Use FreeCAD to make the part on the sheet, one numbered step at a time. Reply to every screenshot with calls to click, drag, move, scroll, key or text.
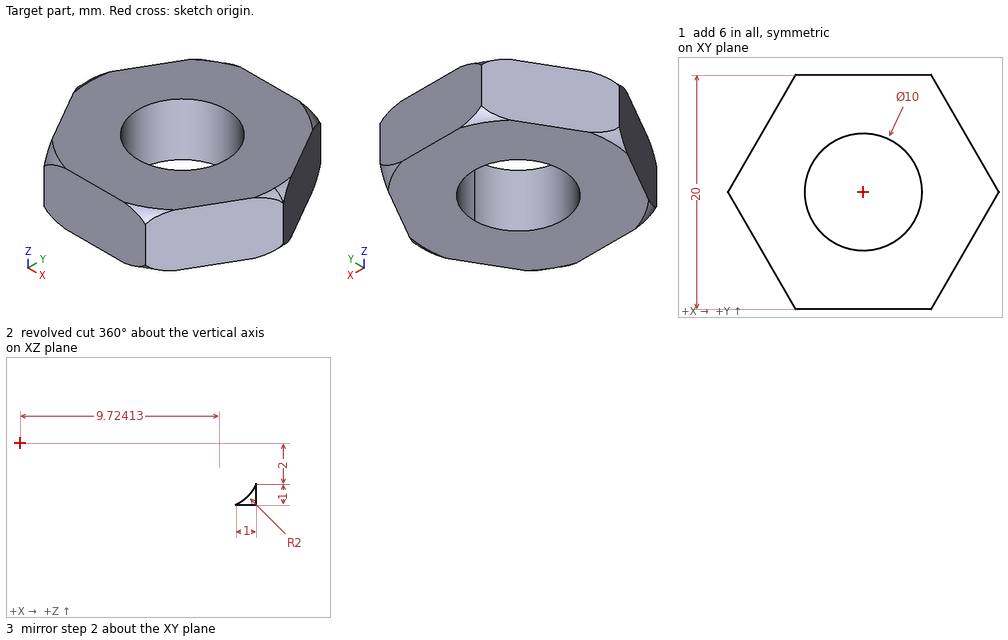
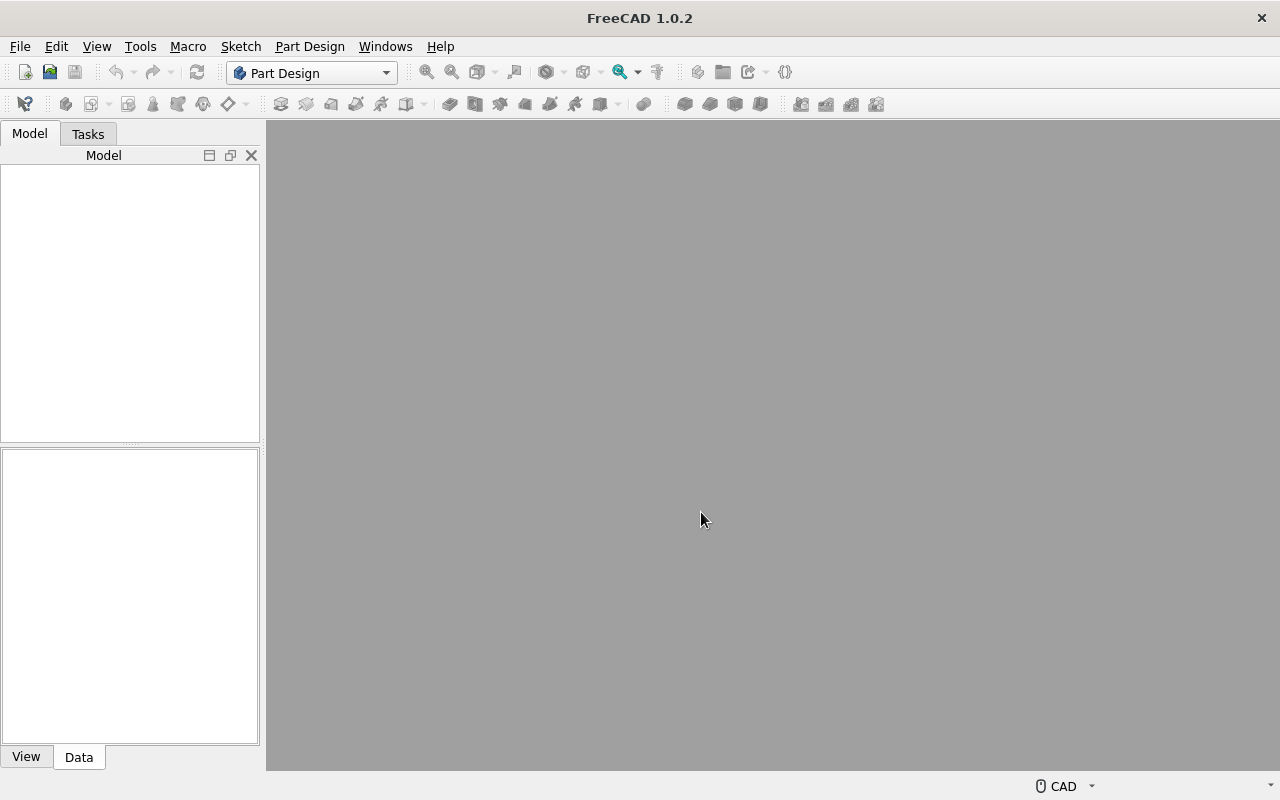
click(25, 72)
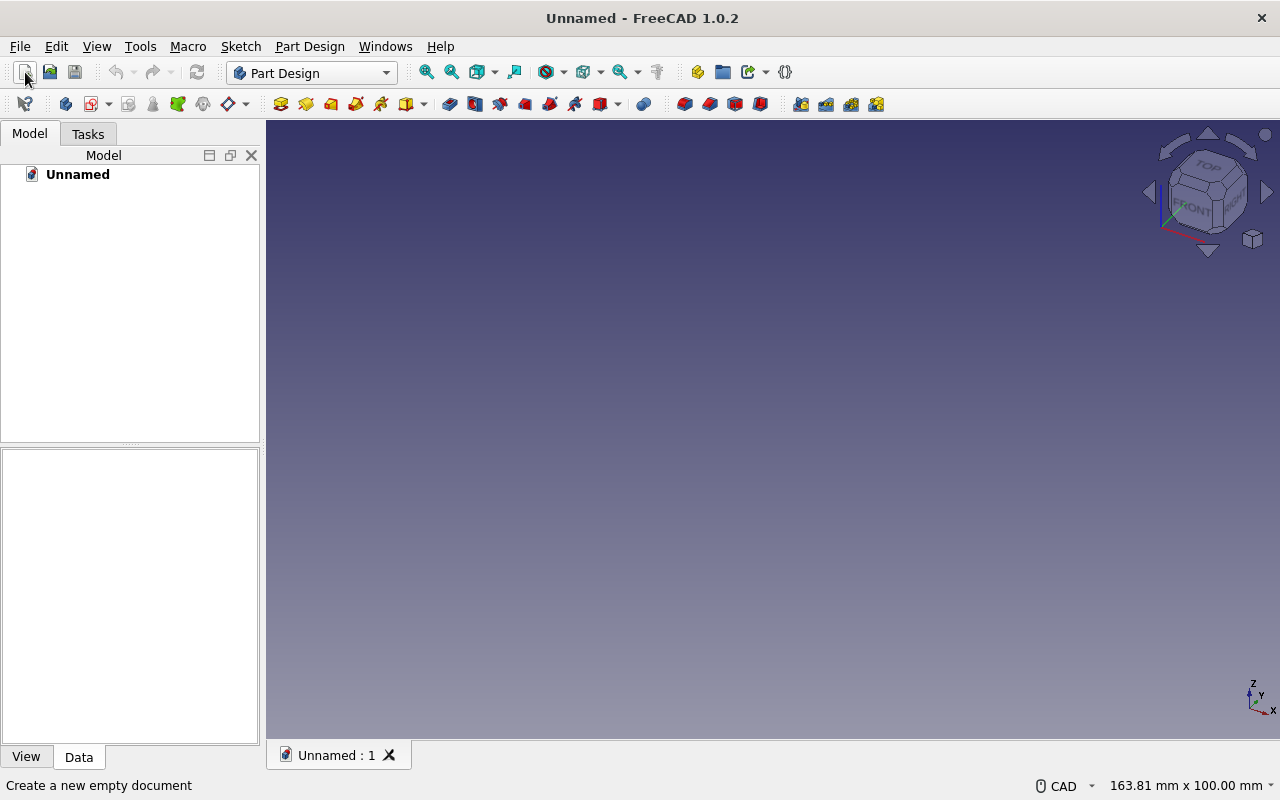
click(90, 104)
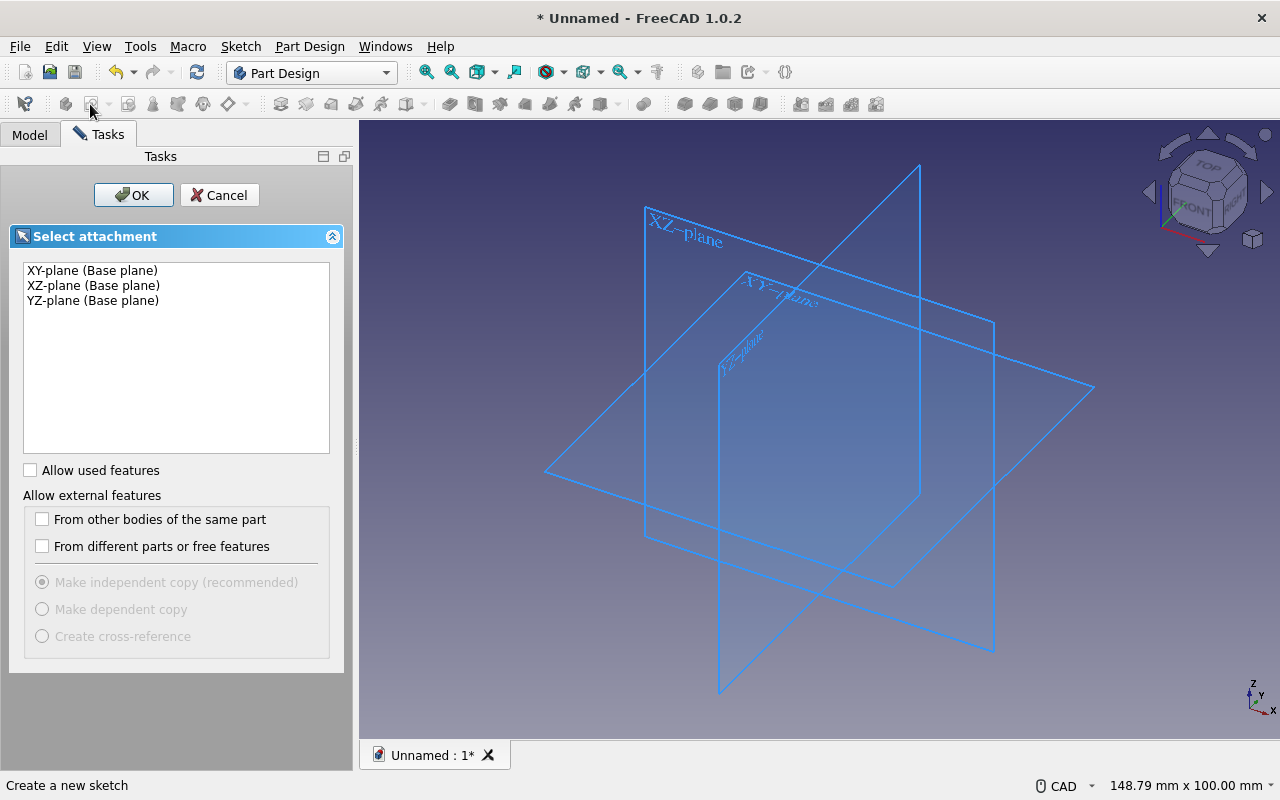
click(84, 270)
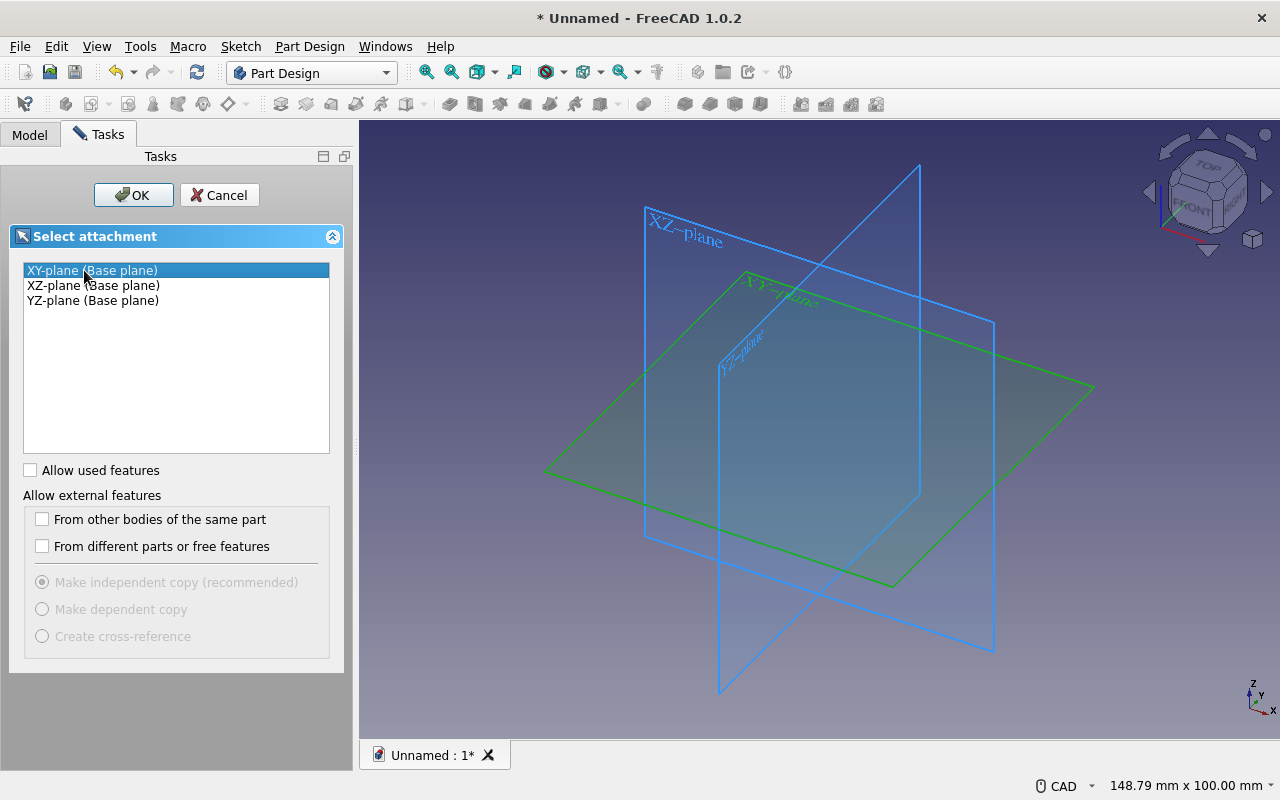
click(134, 195)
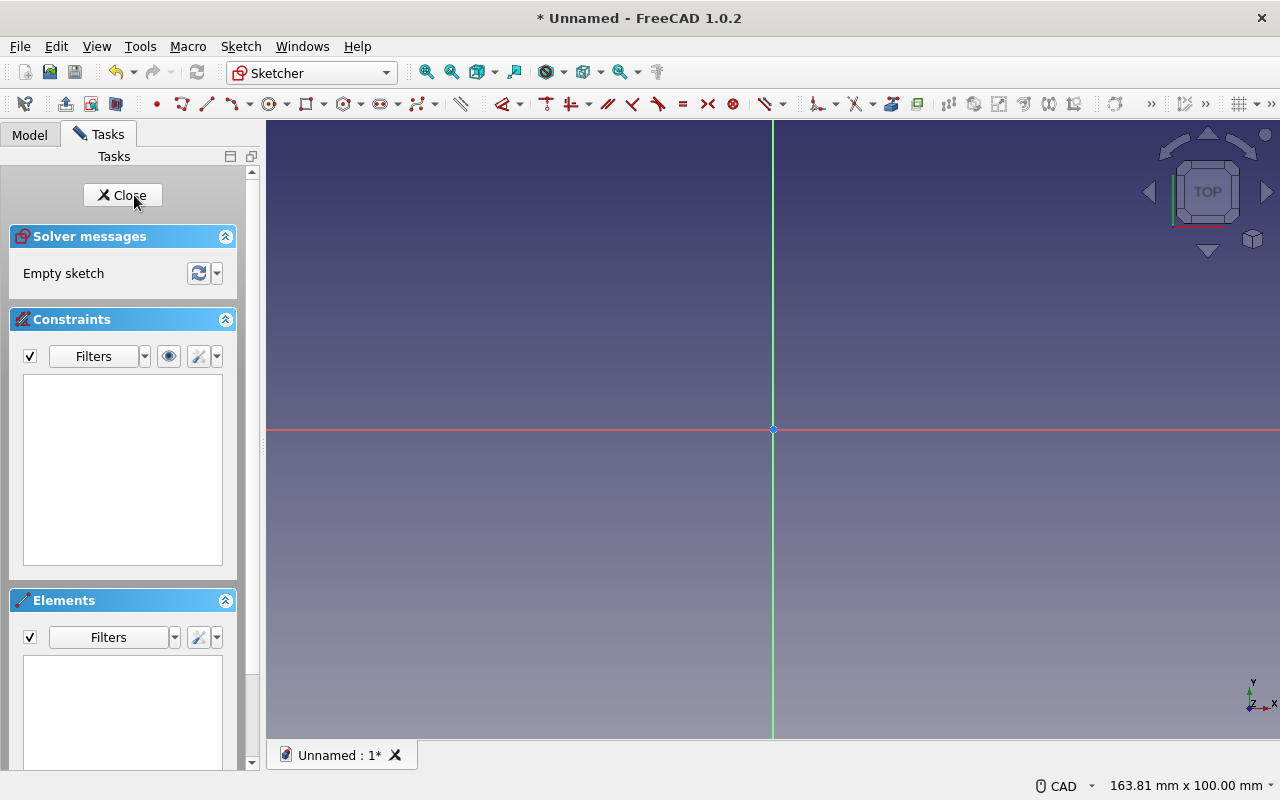
scroll(803, 430, up, 6)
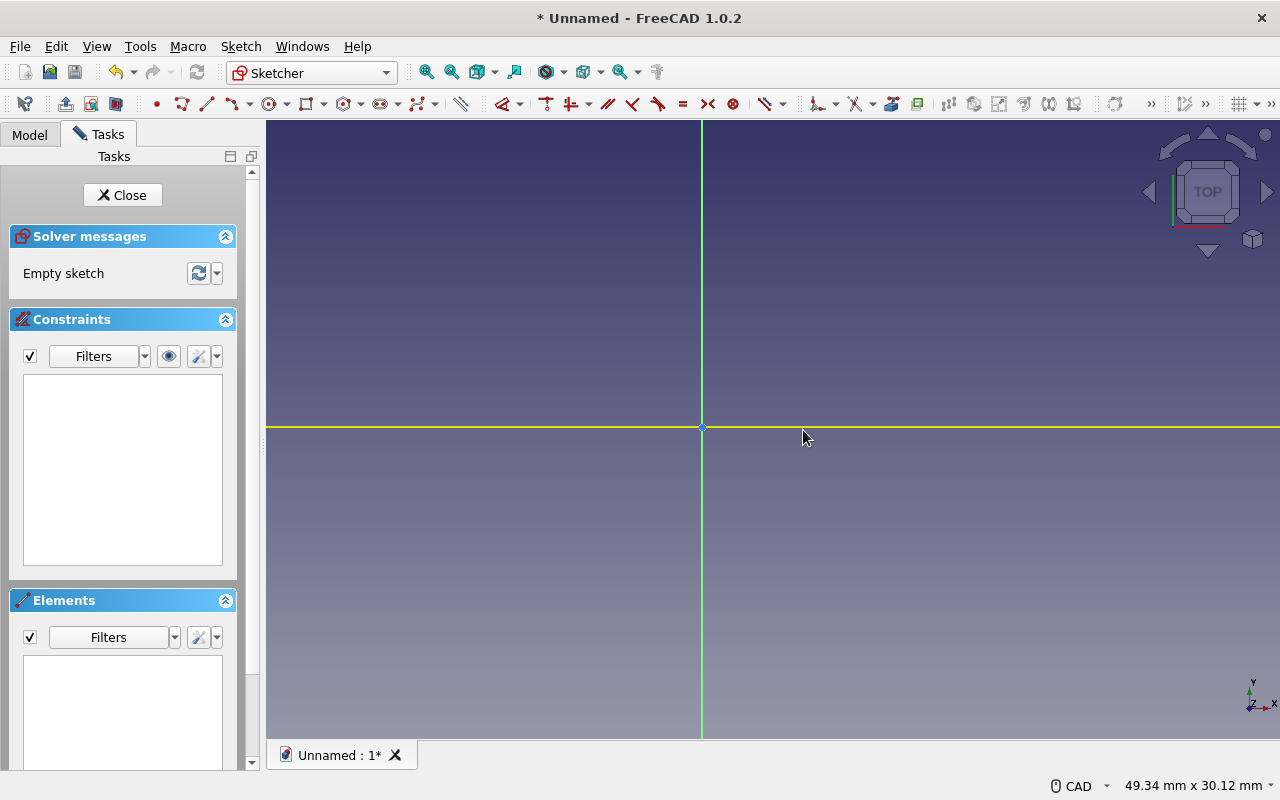
key(g)
key(p)
key(6)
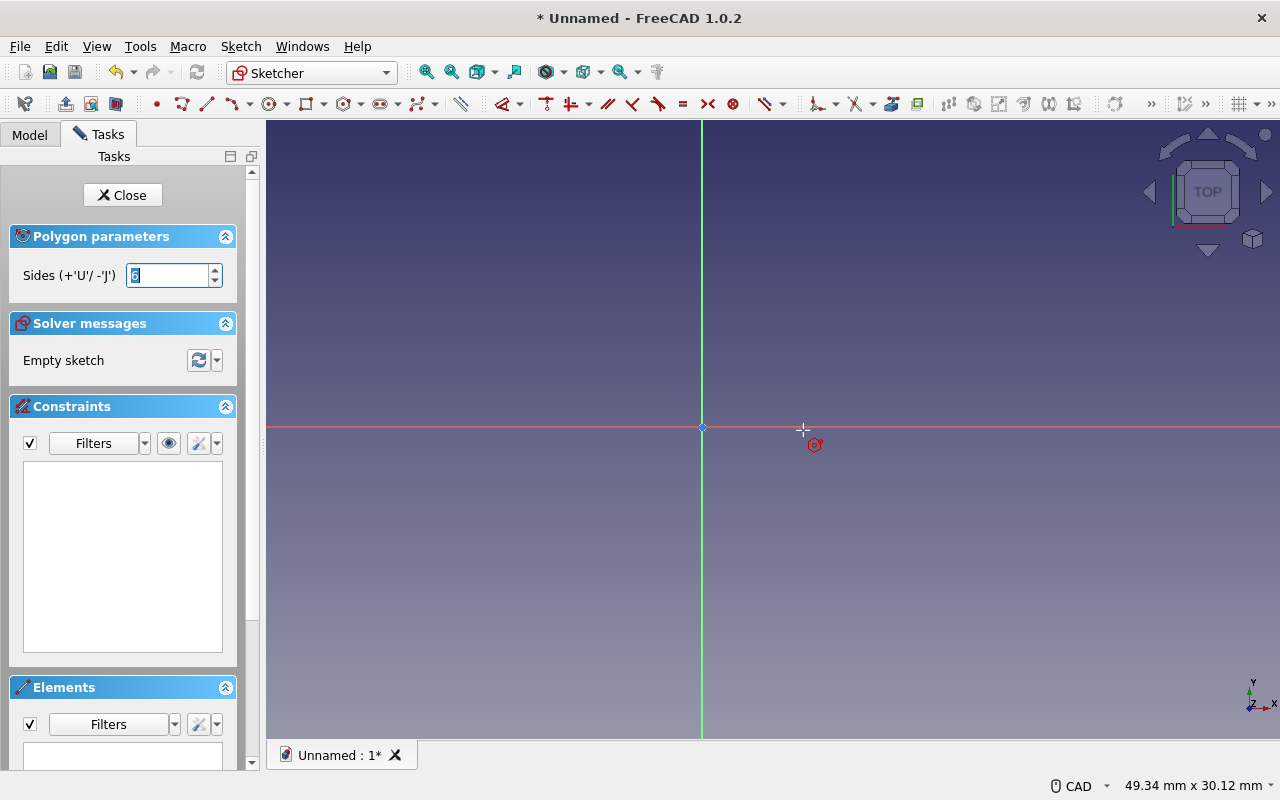
click(702, 427)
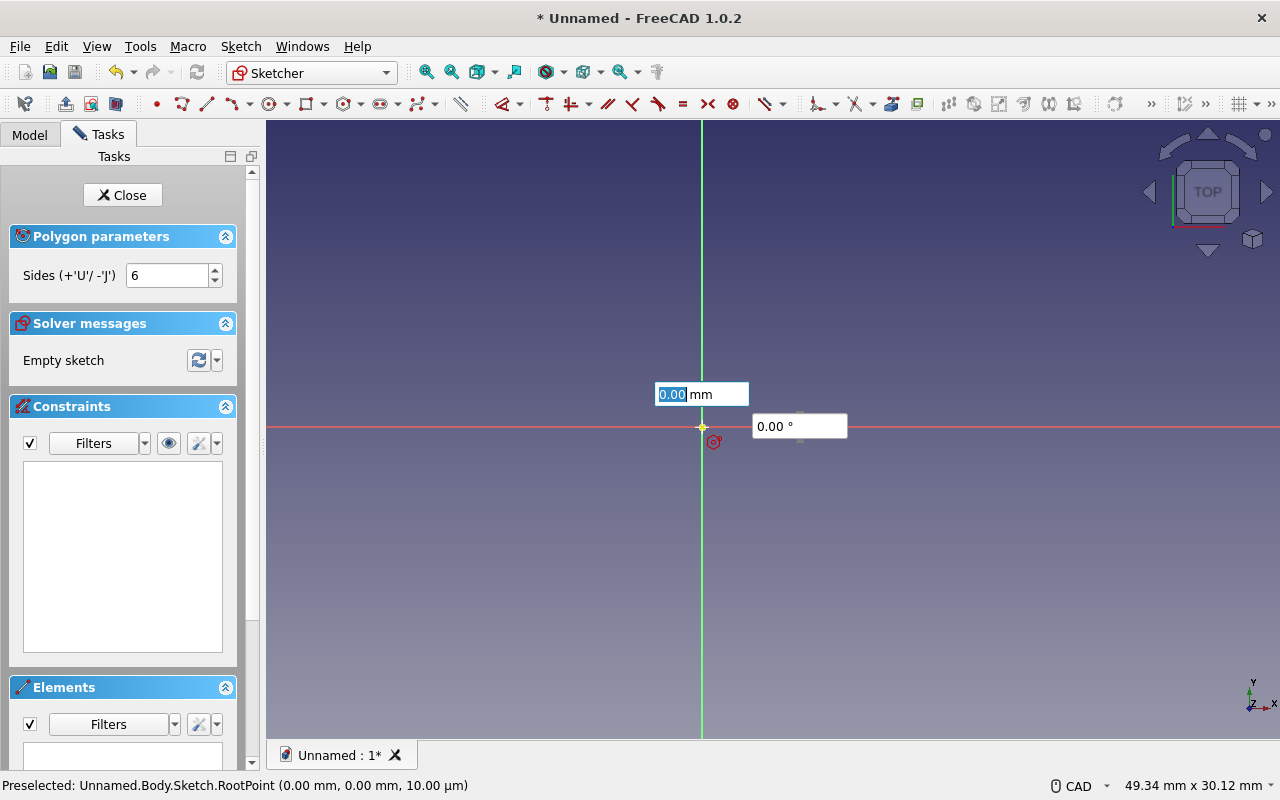
click(939, 427)
right_click(939, 427)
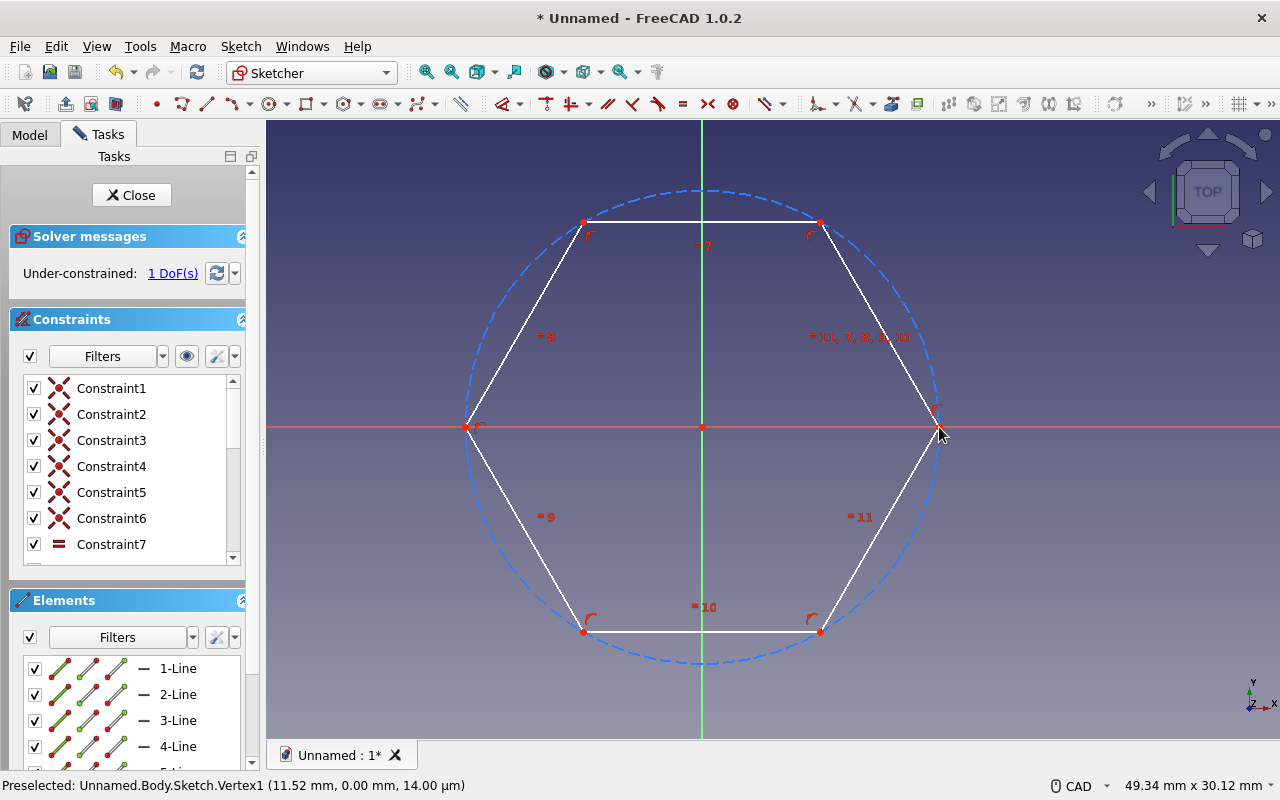
key(g)
key(c)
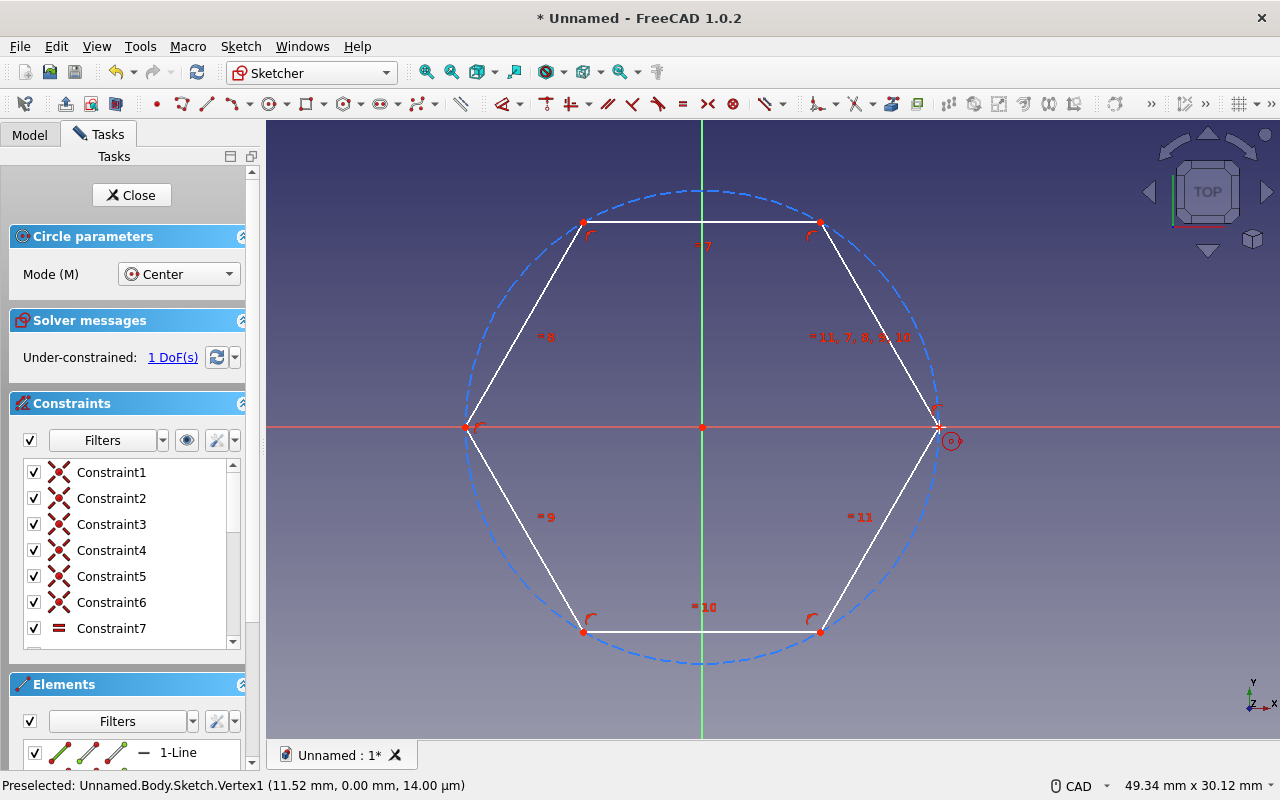
click(702, 427)
click(775, 355)
key(Escape)